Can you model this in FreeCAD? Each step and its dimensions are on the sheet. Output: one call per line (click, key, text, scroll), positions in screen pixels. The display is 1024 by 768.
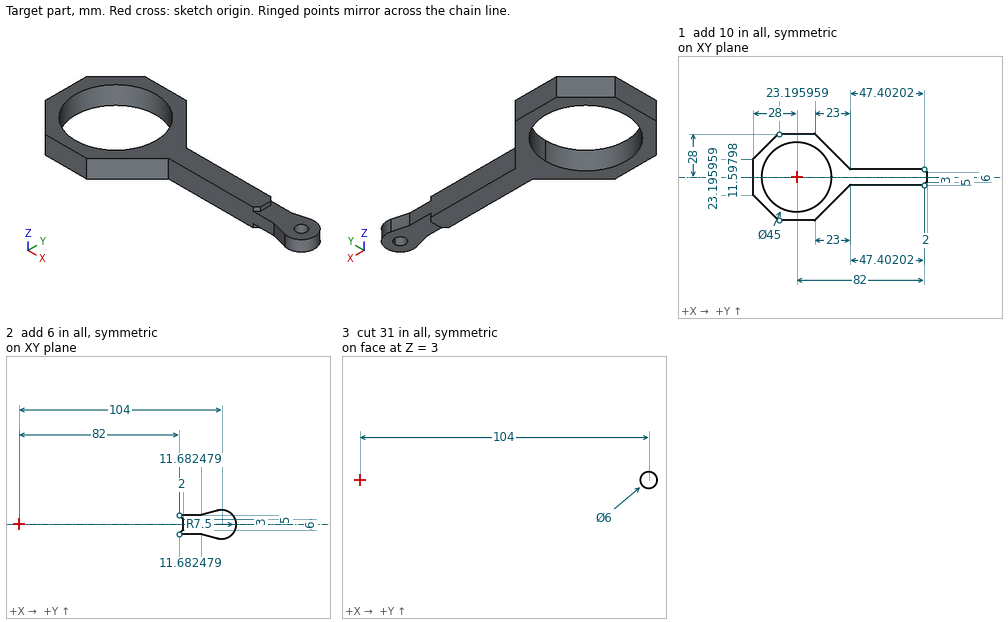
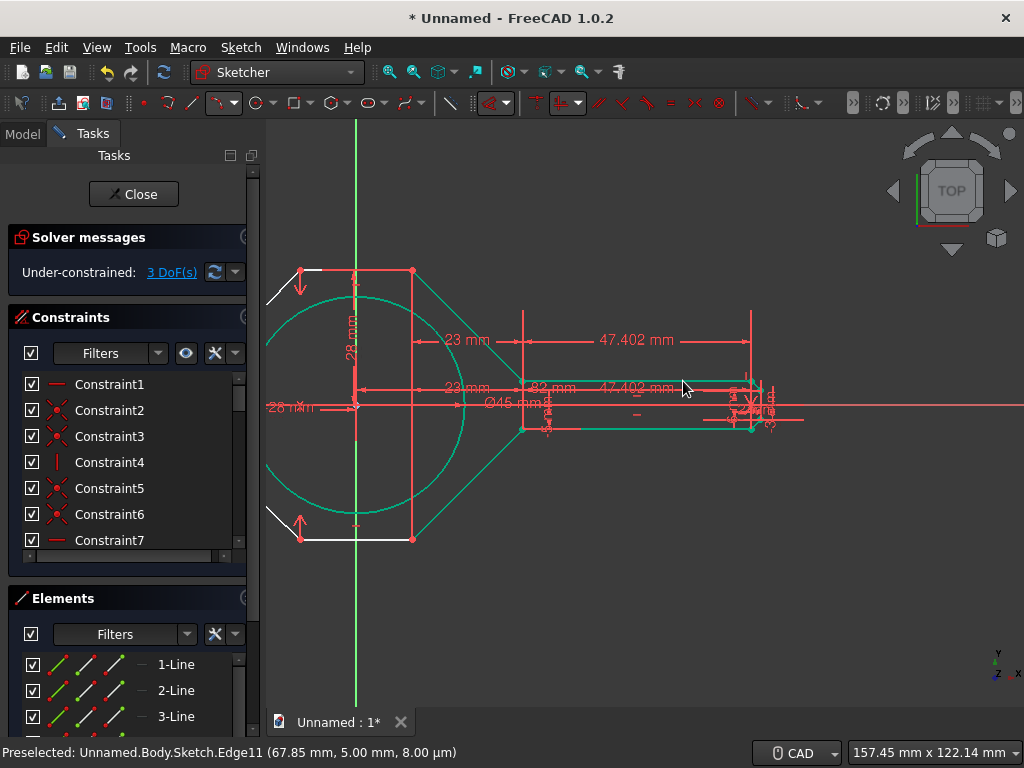
click(379, 270)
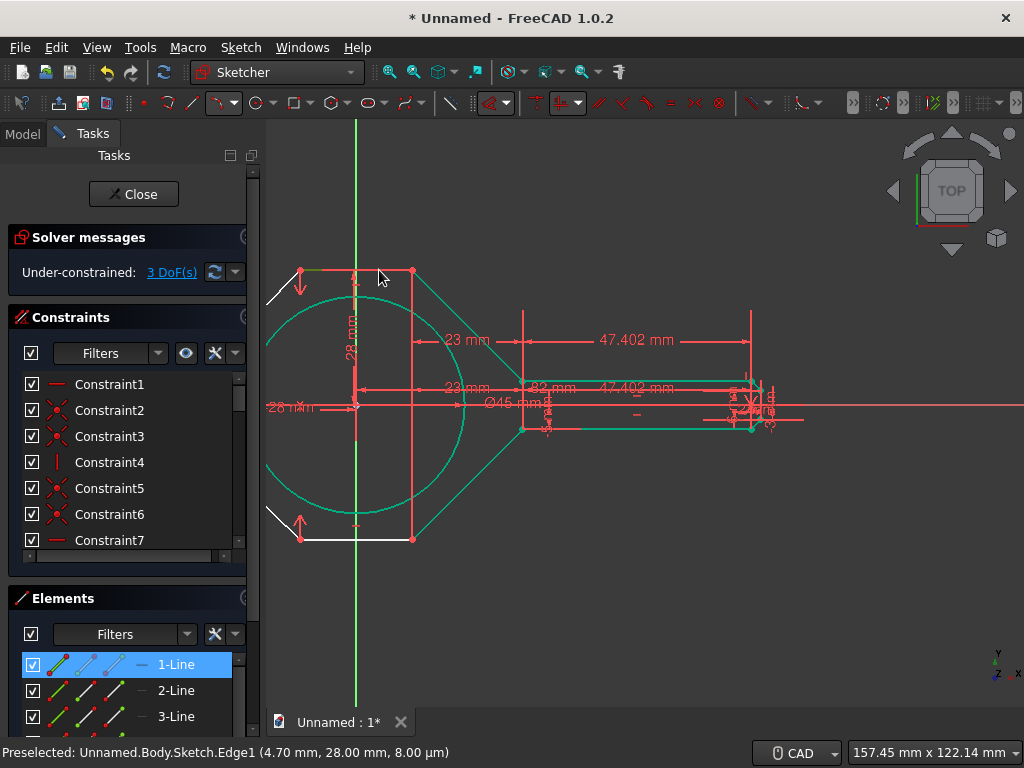
click(508, 104)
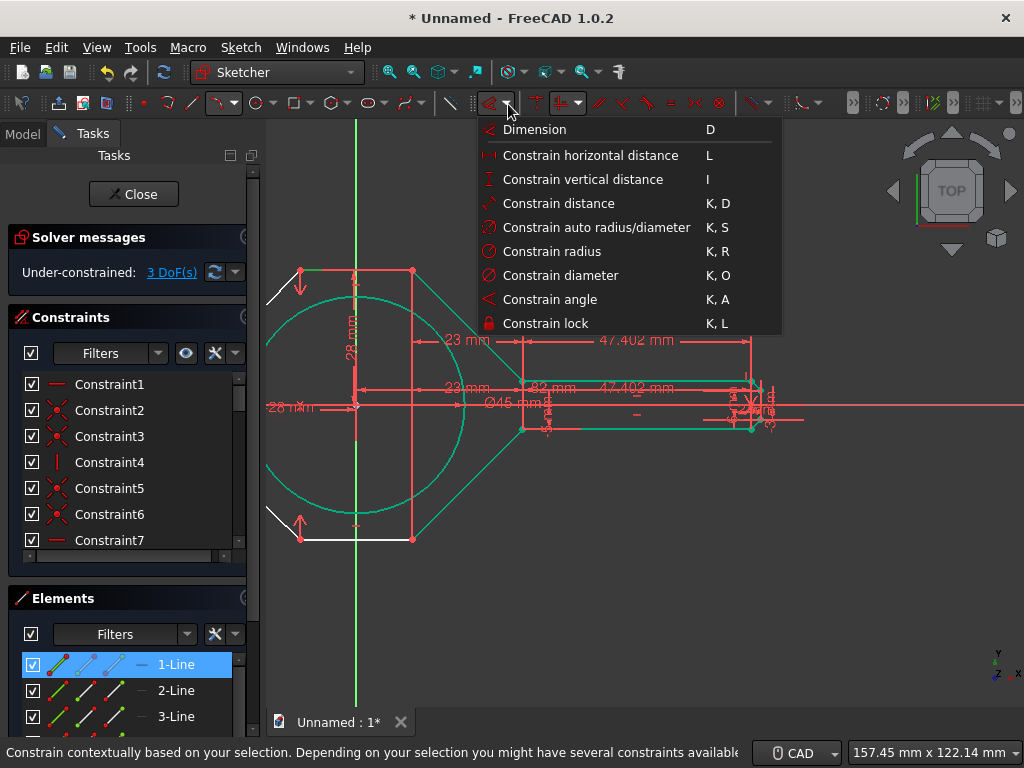
click(630, 155)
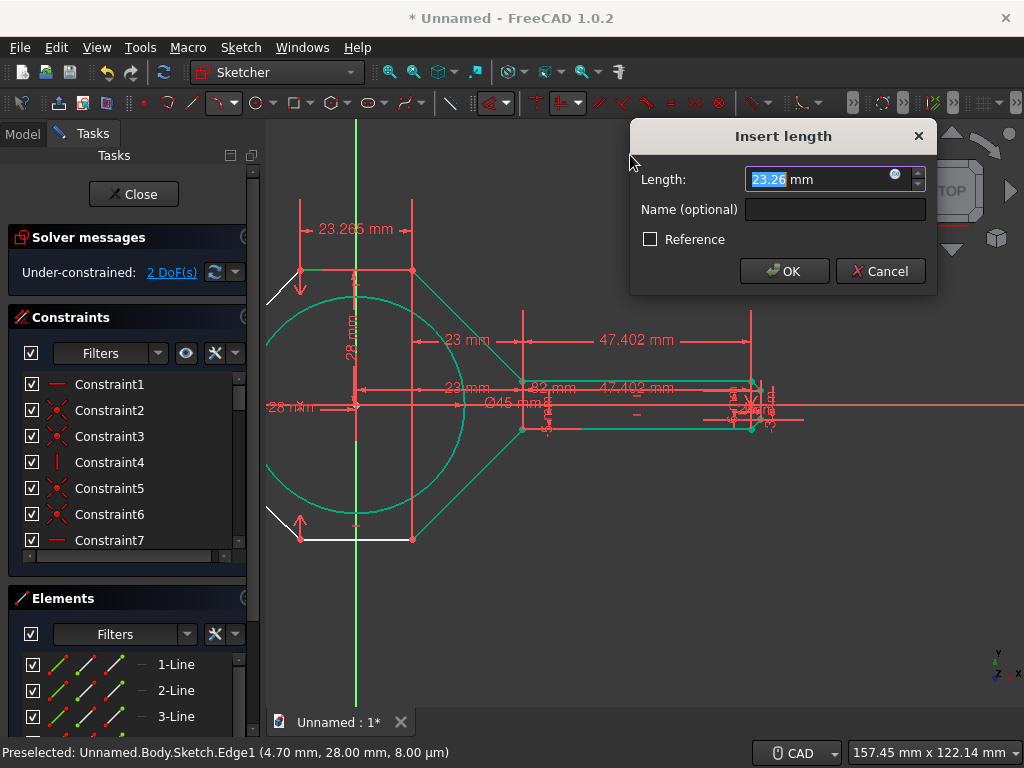
text(23.195959)
key(Return)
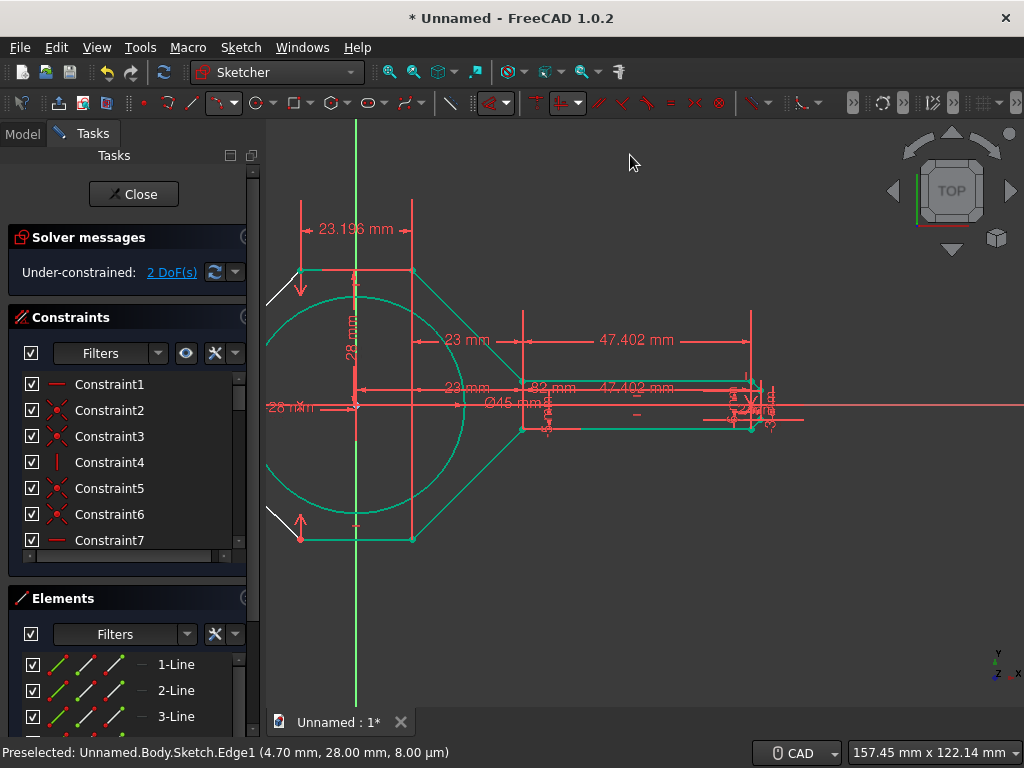
scroll(750, 429, down, 2)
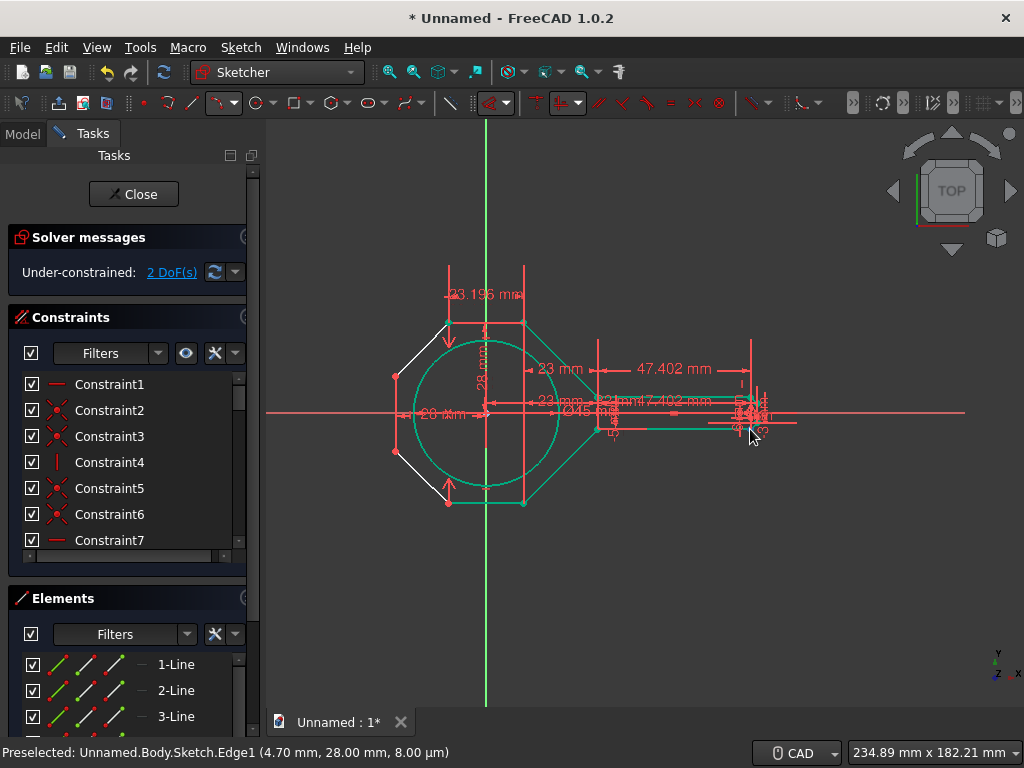
click(396, 399)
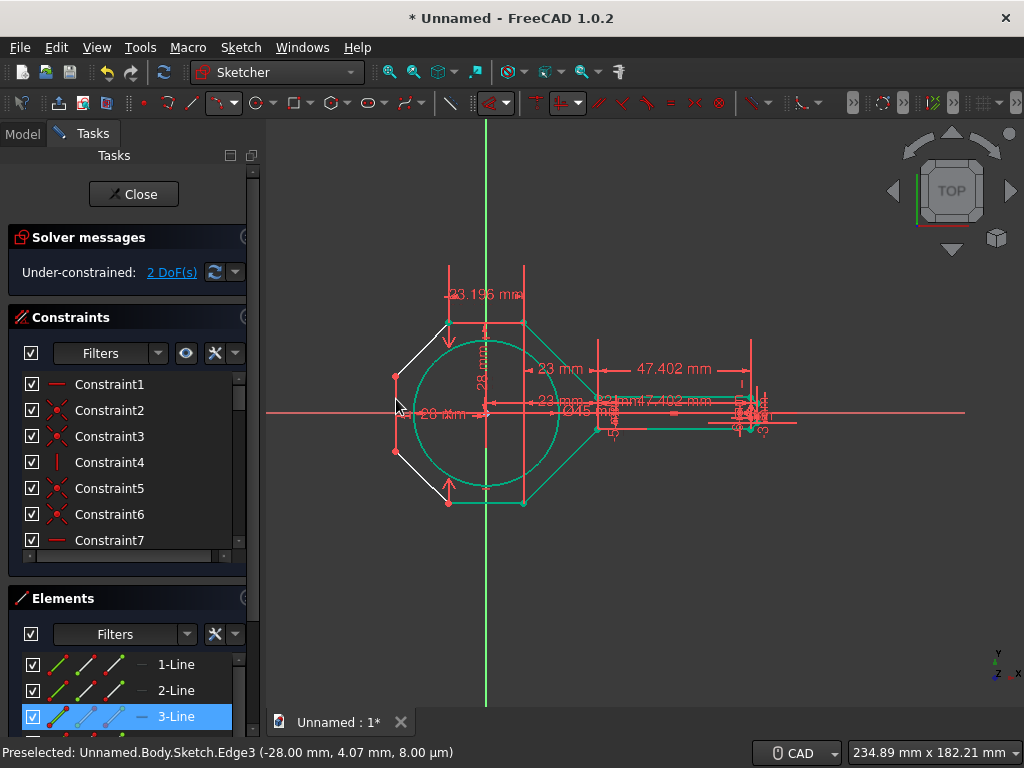
click(508, 104)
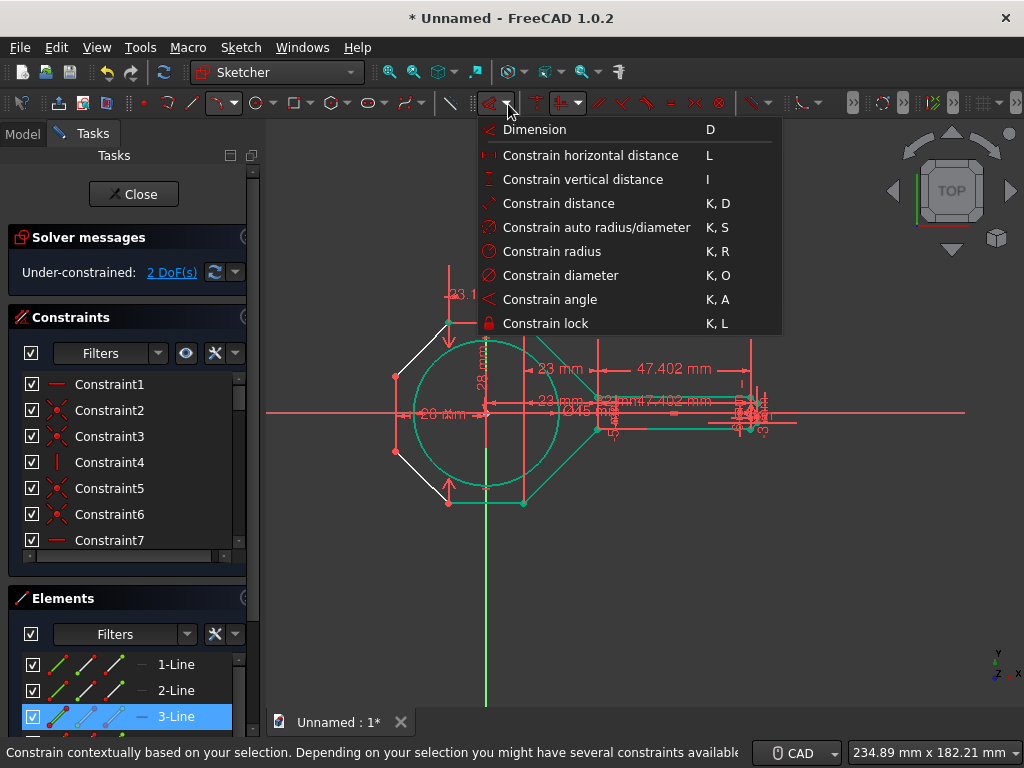
click(630, 179)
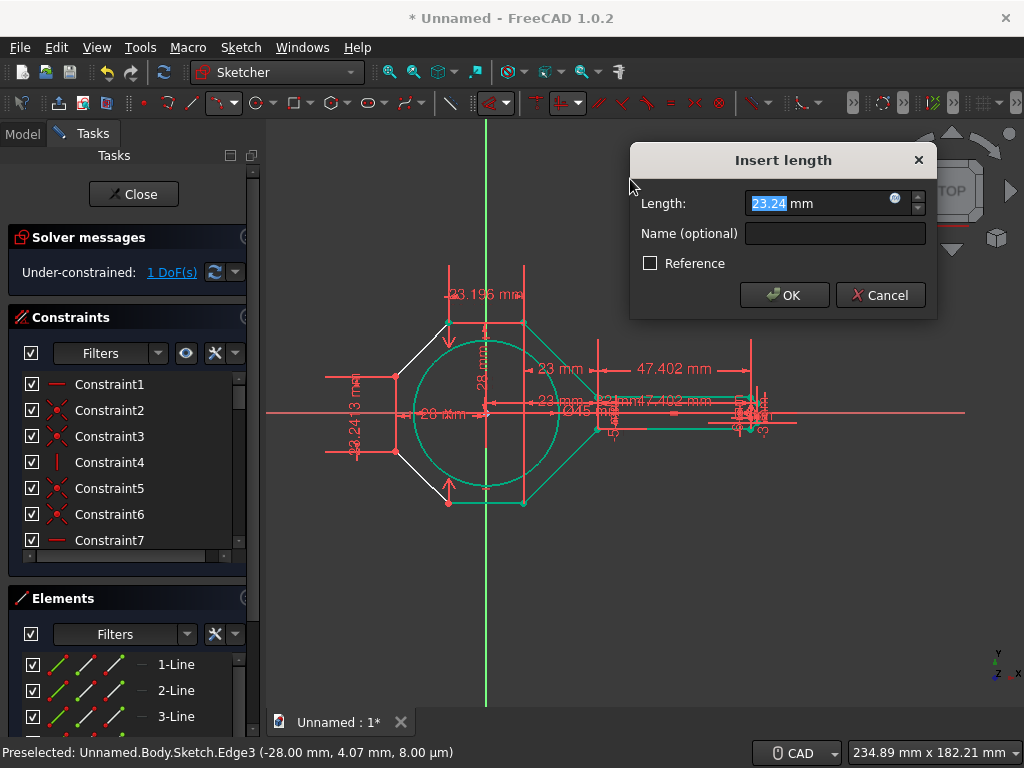
text(23.195959)
key(Return)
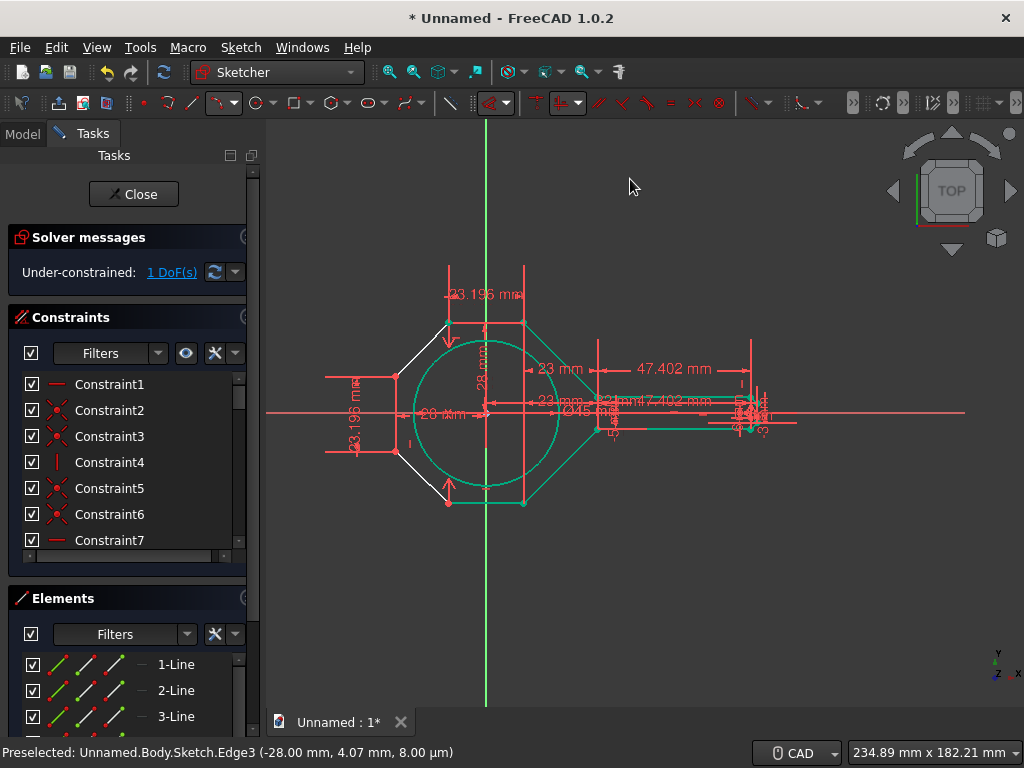
click(396, 377)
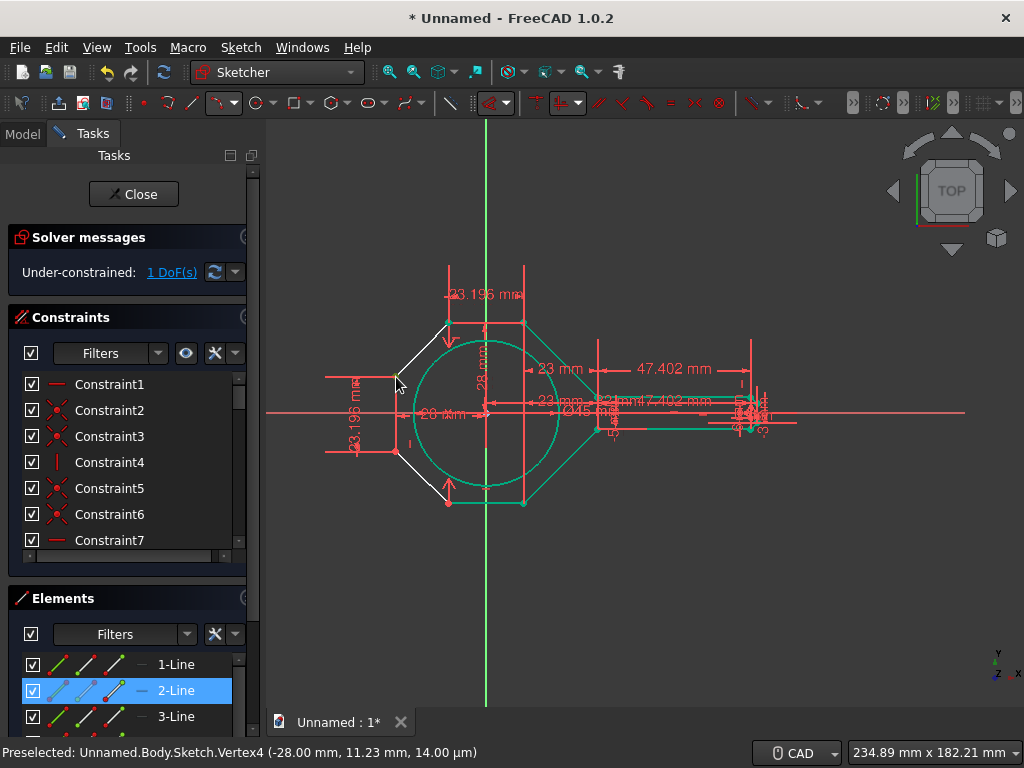
key(i)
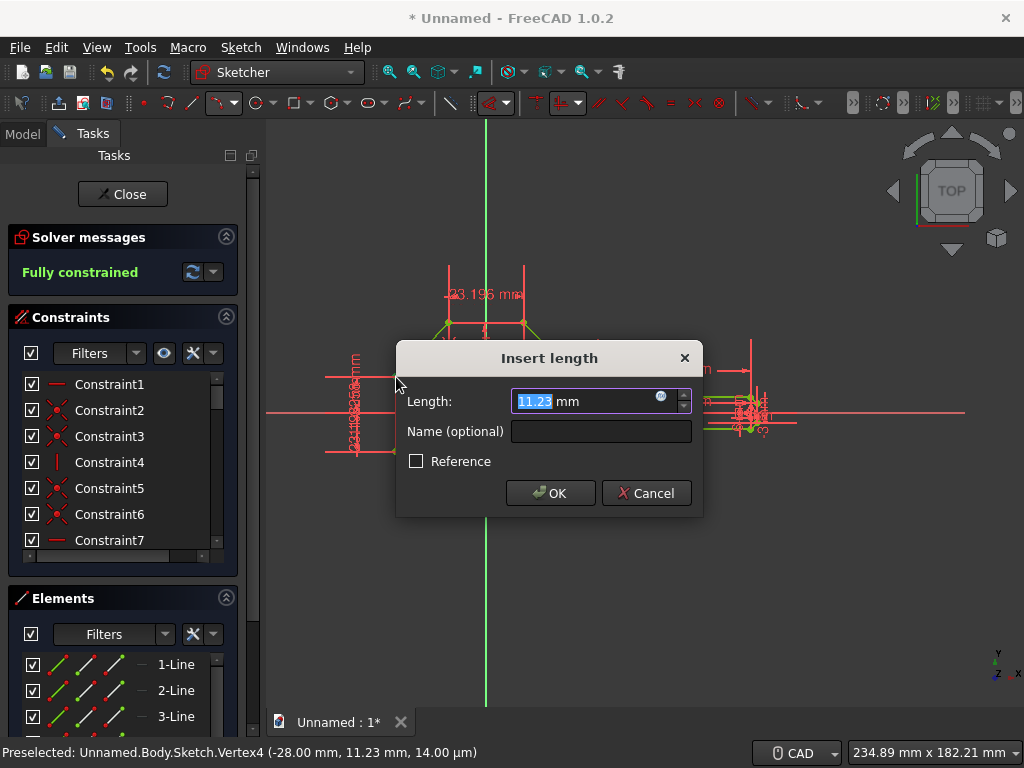
text(11.59798)
key(Return)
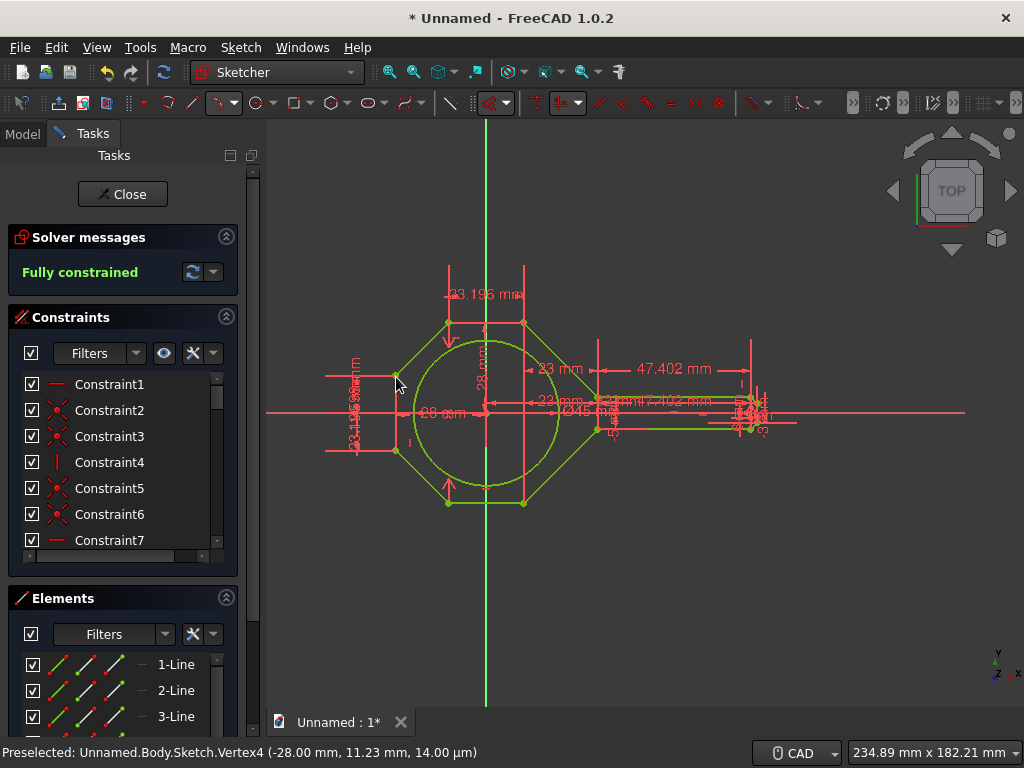
click(123, 194)